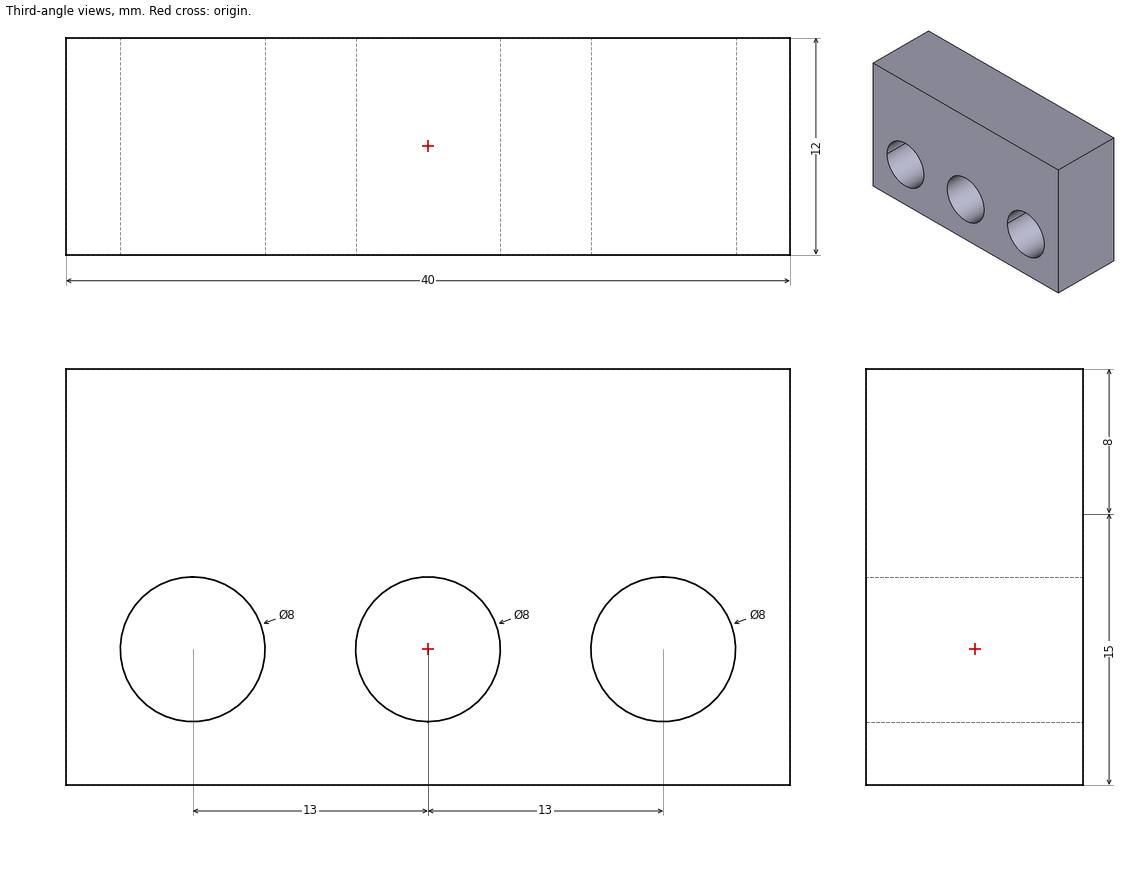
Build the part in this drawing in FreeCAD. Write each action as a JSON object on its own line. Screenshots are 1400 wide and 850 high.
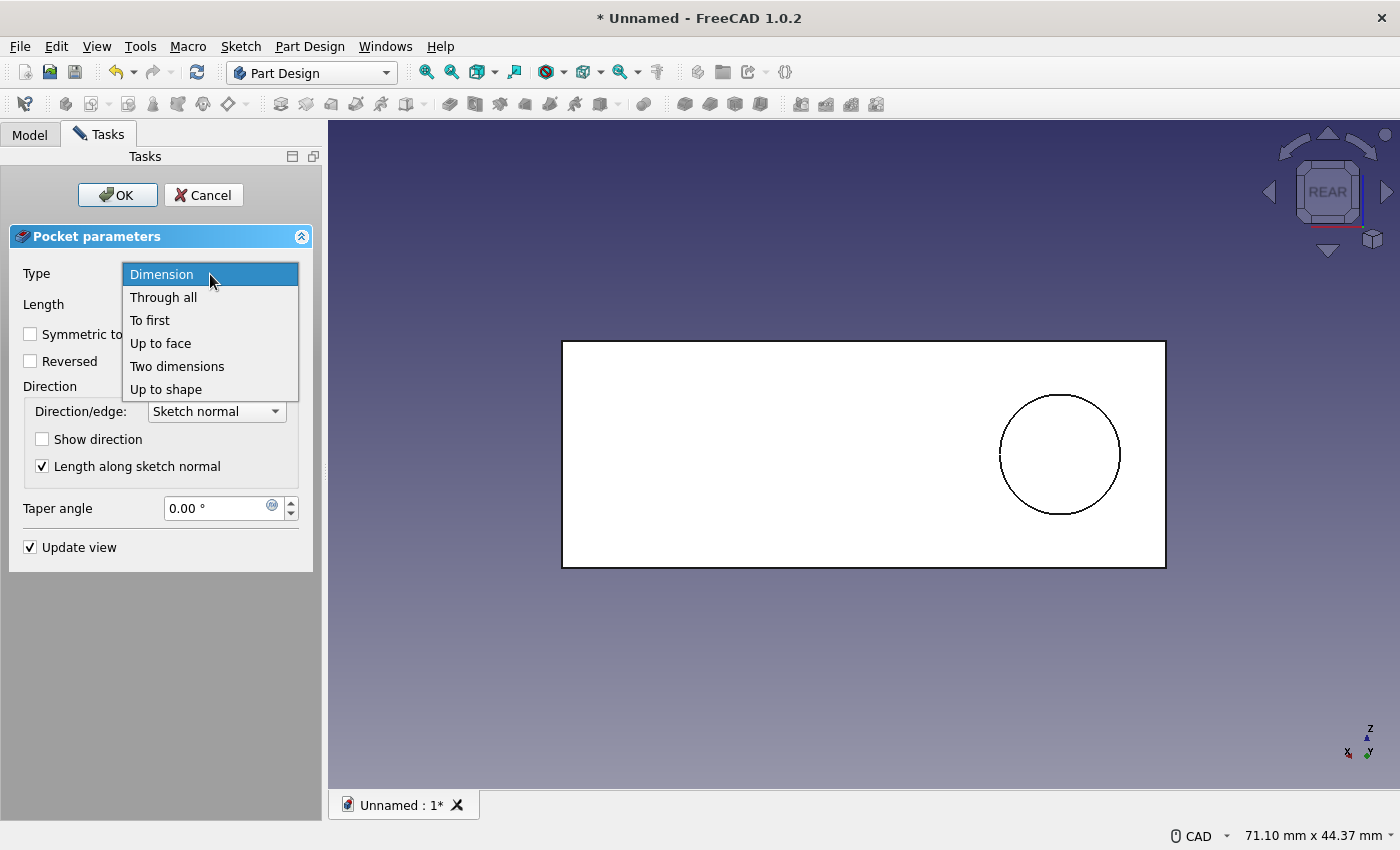
{"action": "left_click", "coordinate": [208, 320]}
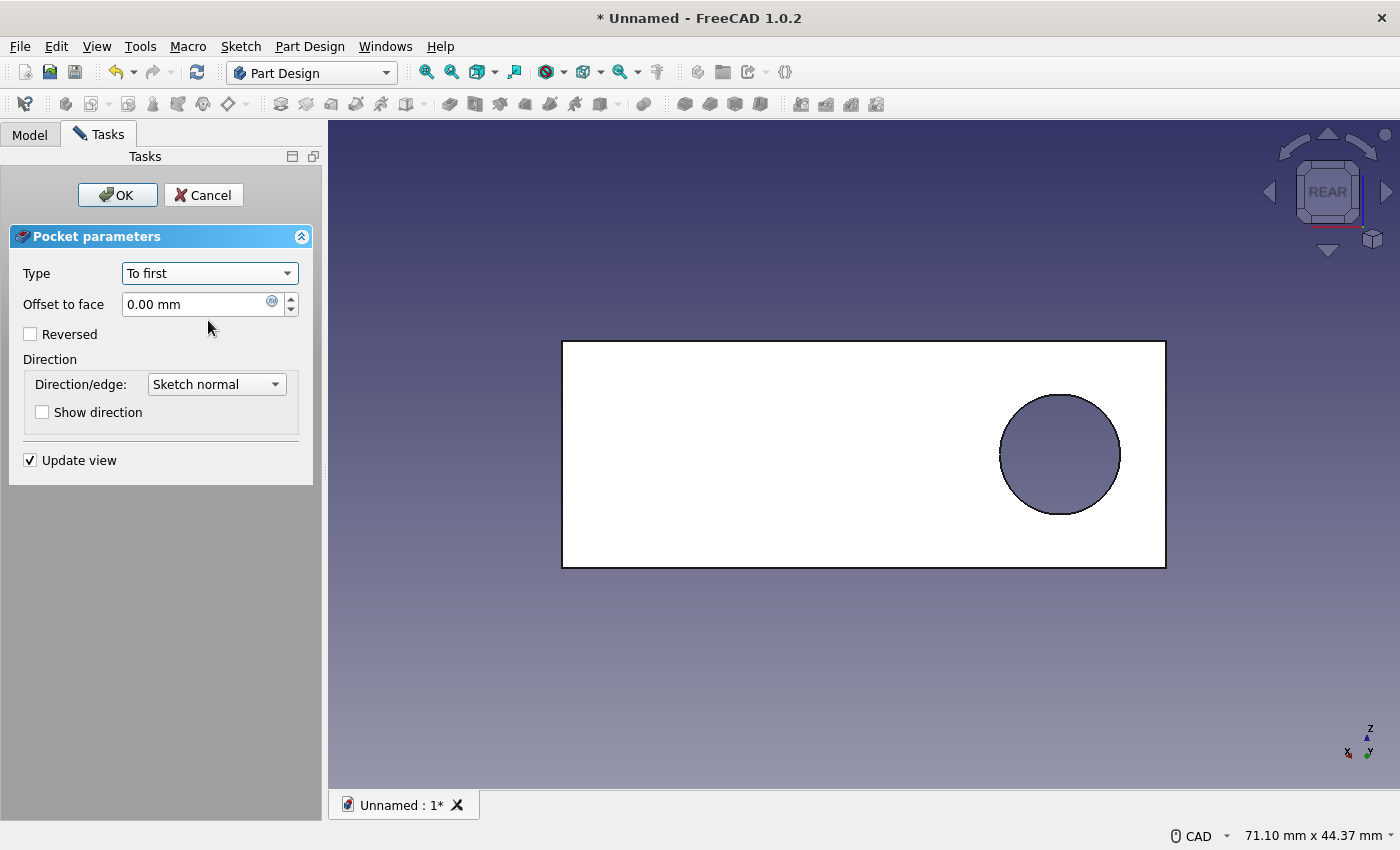
{"action": "left_click", "coordinate": [118, 195]}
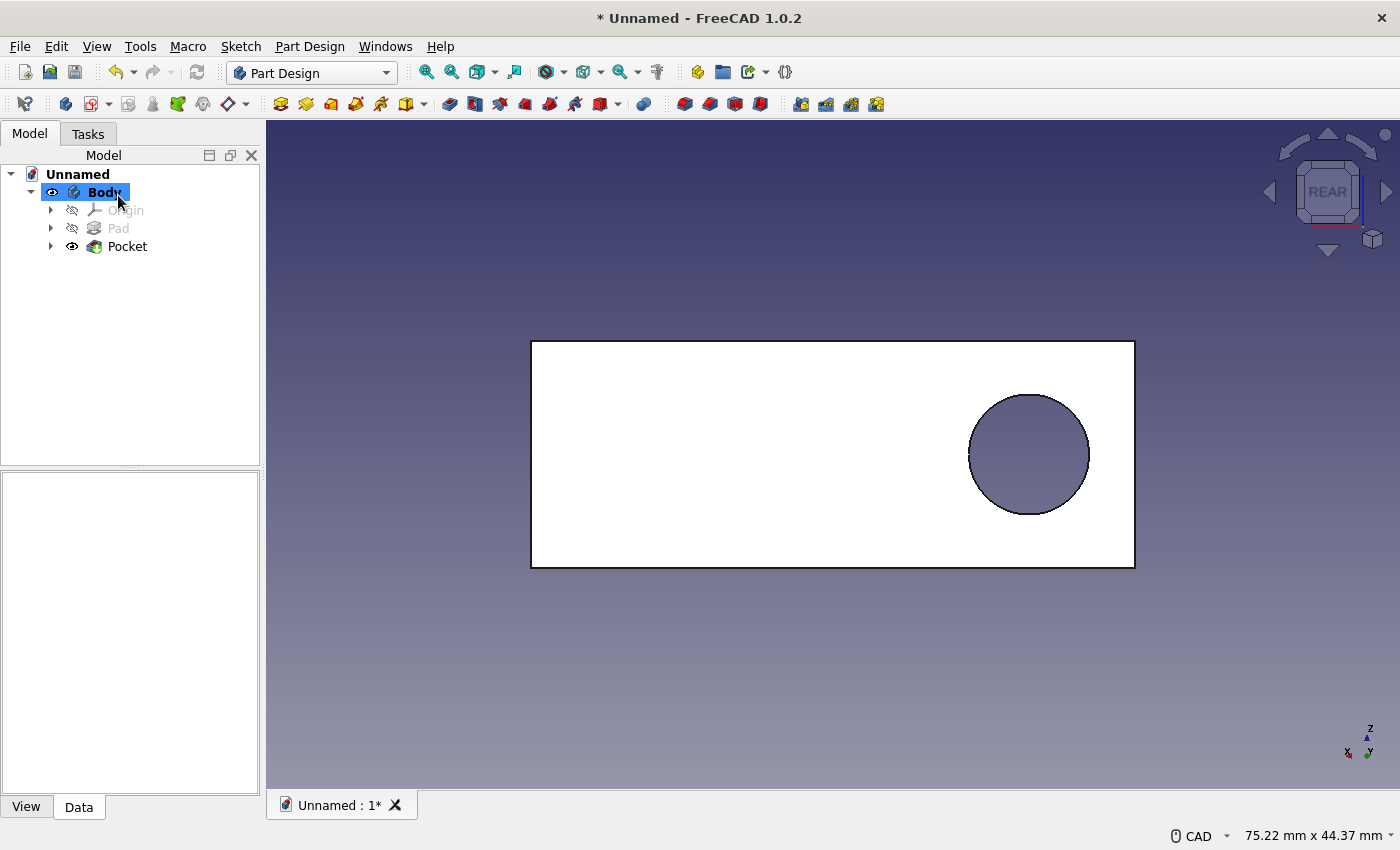
{"action": "left_click", "coordinate": [661, 453]}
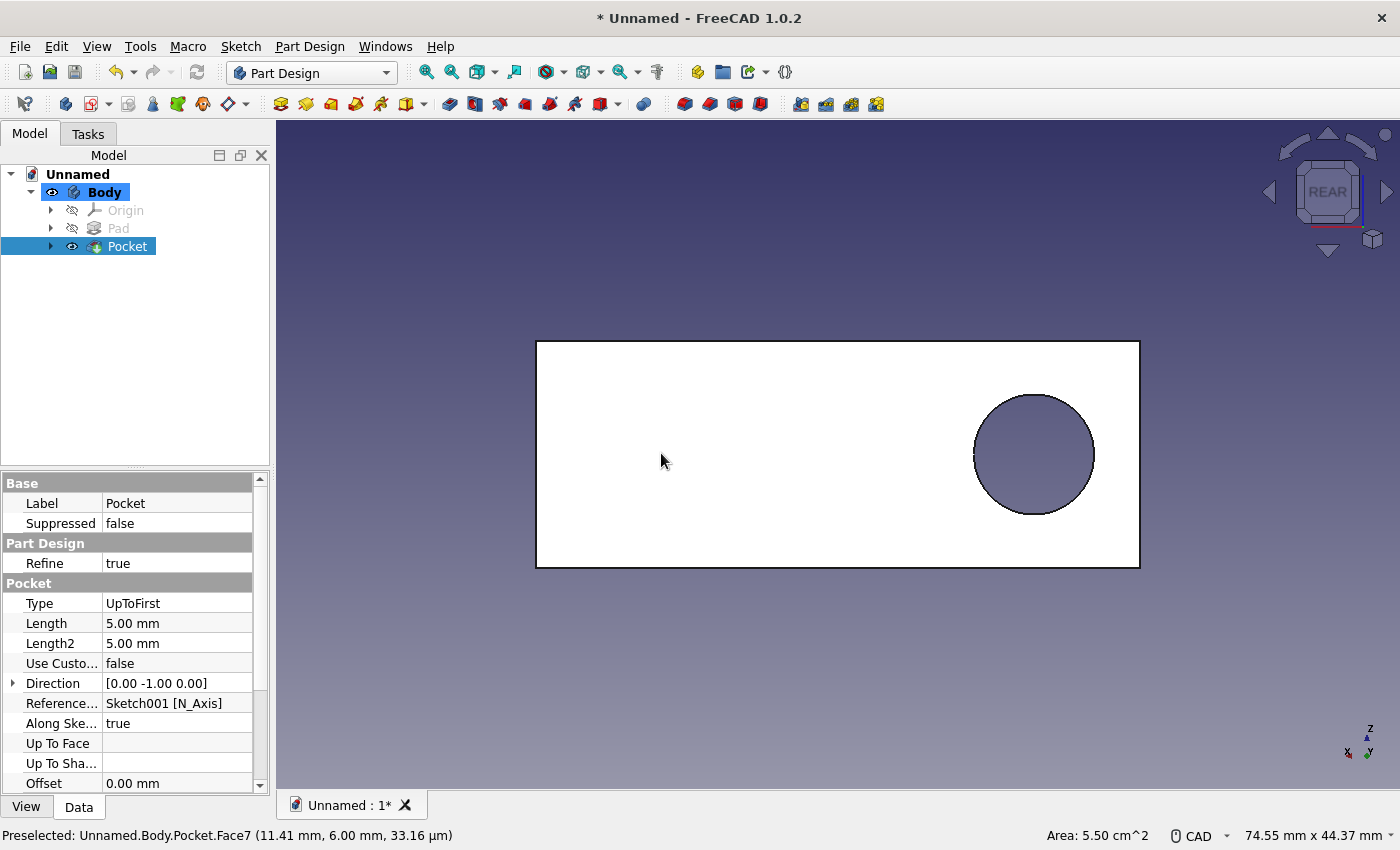
{"action": "left_click", "coordinate": [90, 104]}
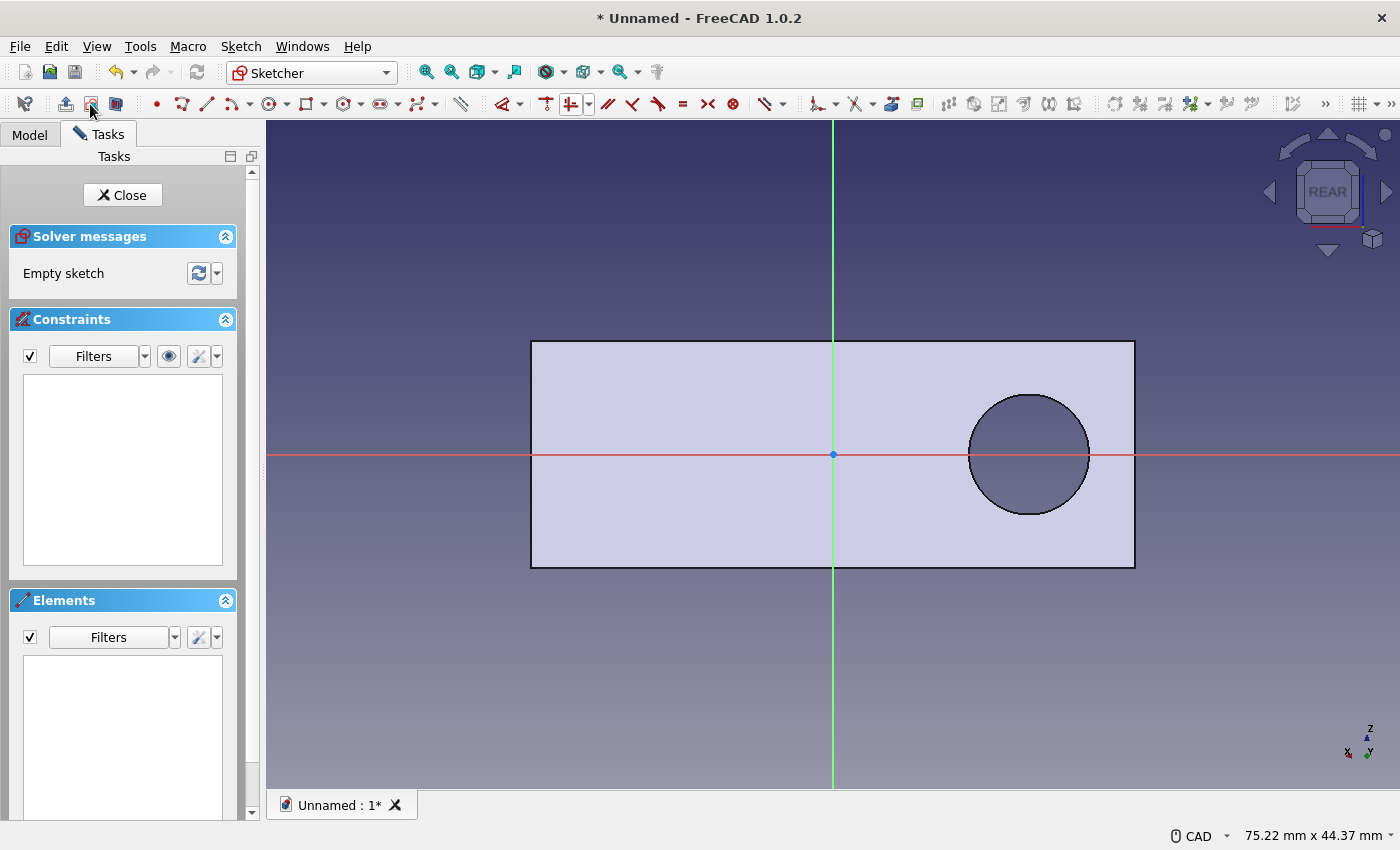
{"action": "scroll", "coordinate": [670, 455], "scroll_direction": "up", "scroll_amount": 5}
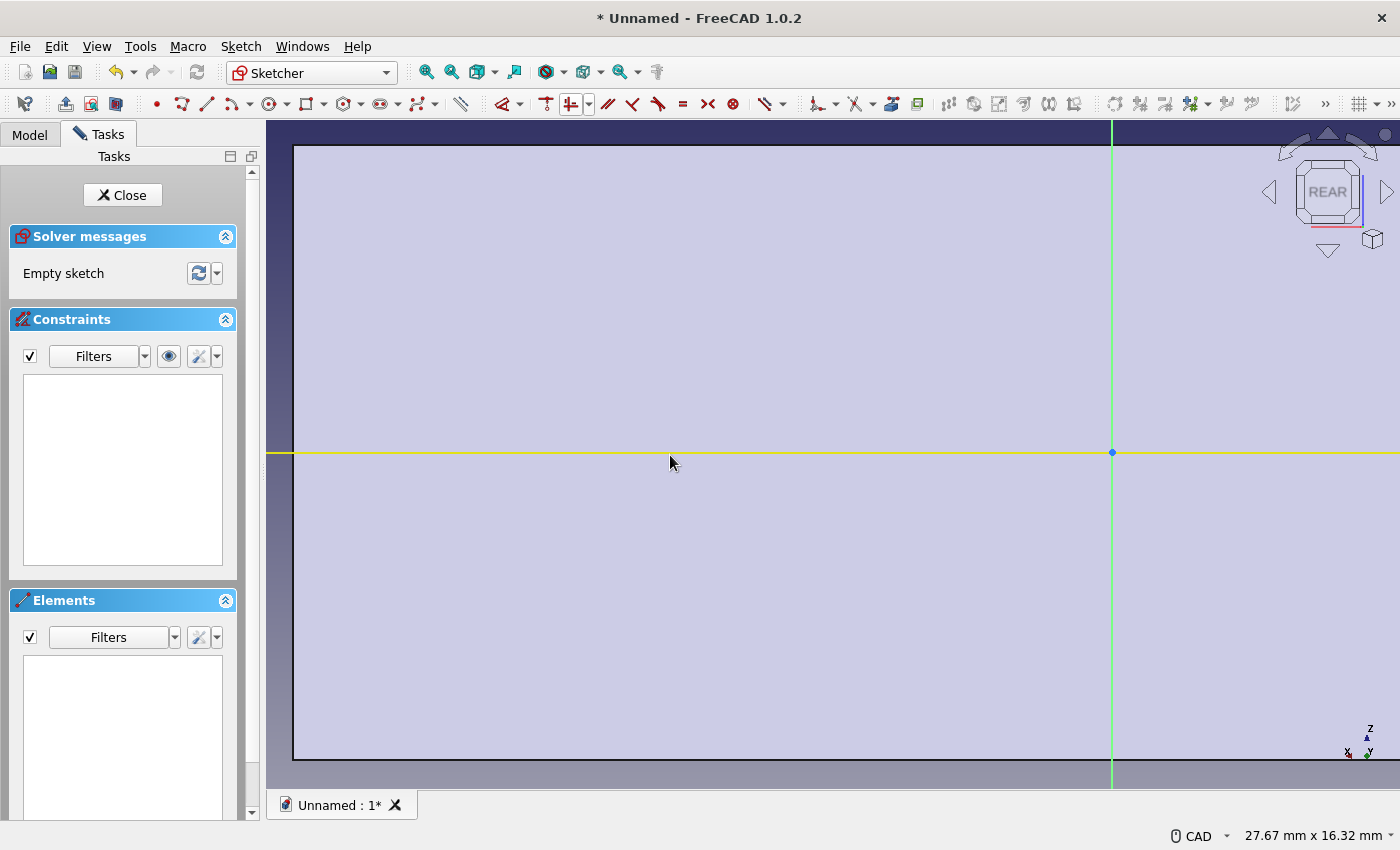
{"action": "left_click", "coordinate": [268, 104]}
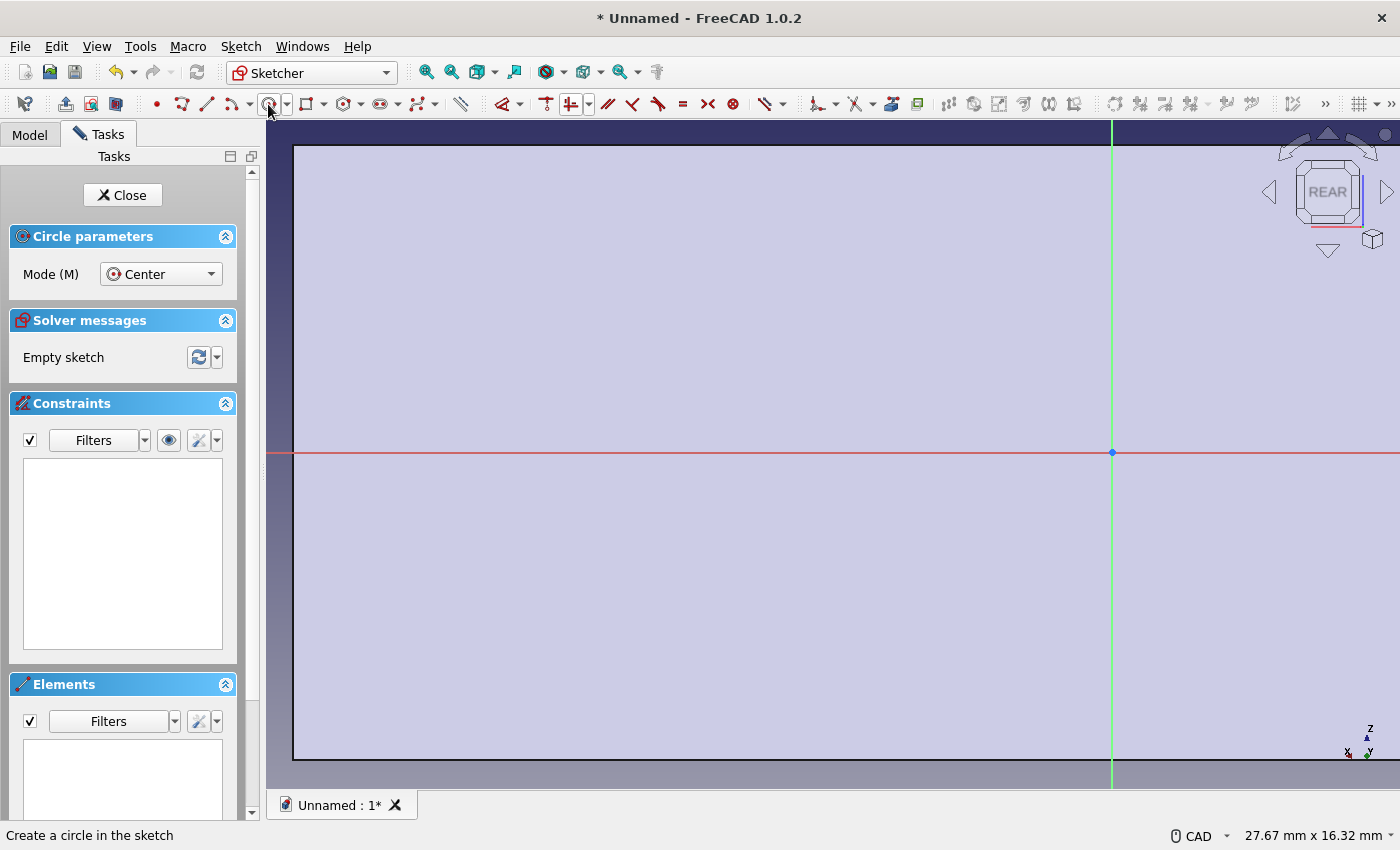
{"action": "left_click", "coordinate": [580, 453]}
{"action": "left_click", "coordinate": [696, 337]}
{"action": "key", "text": "Escape"}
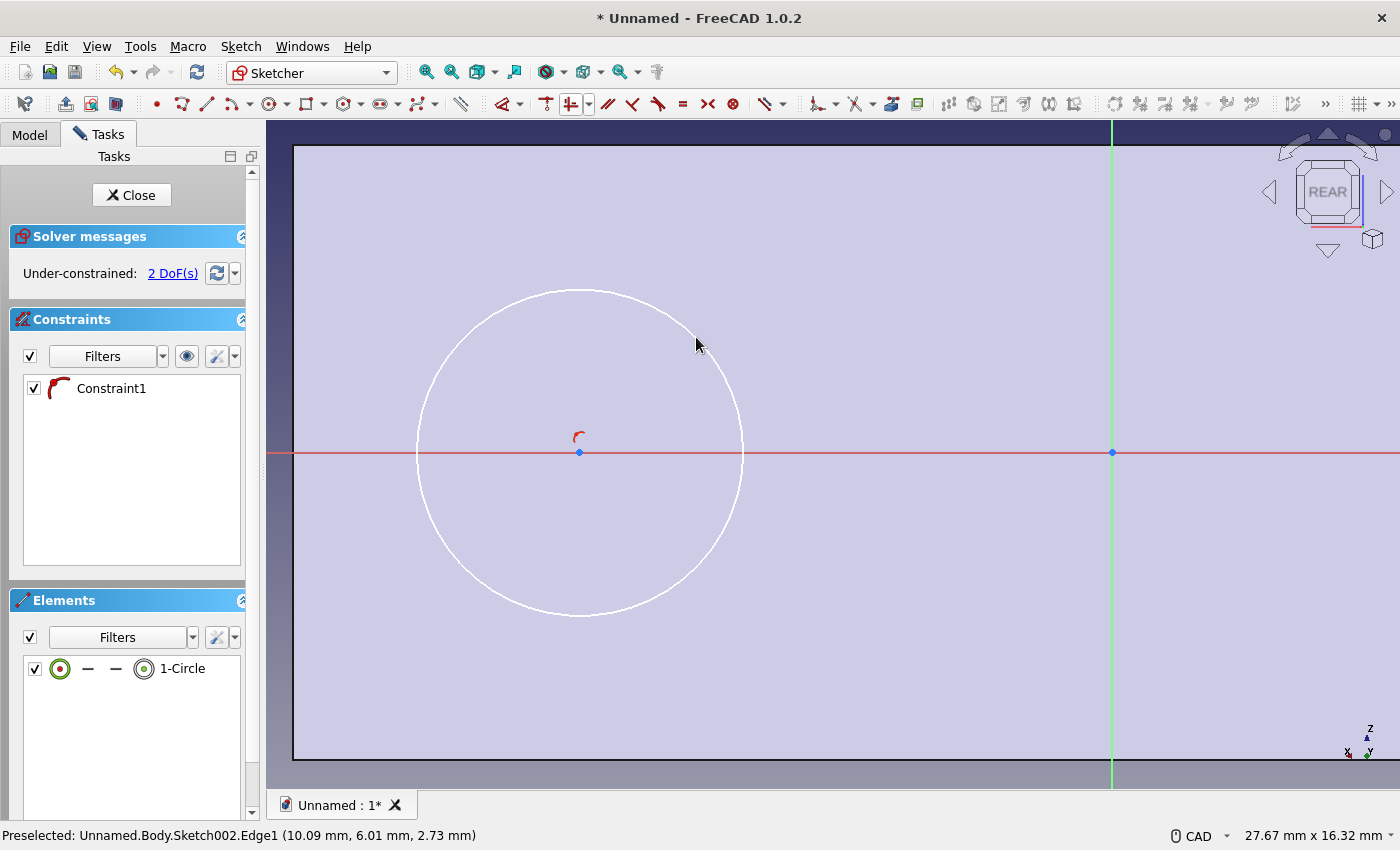
{"action": "key", "text": "d"}